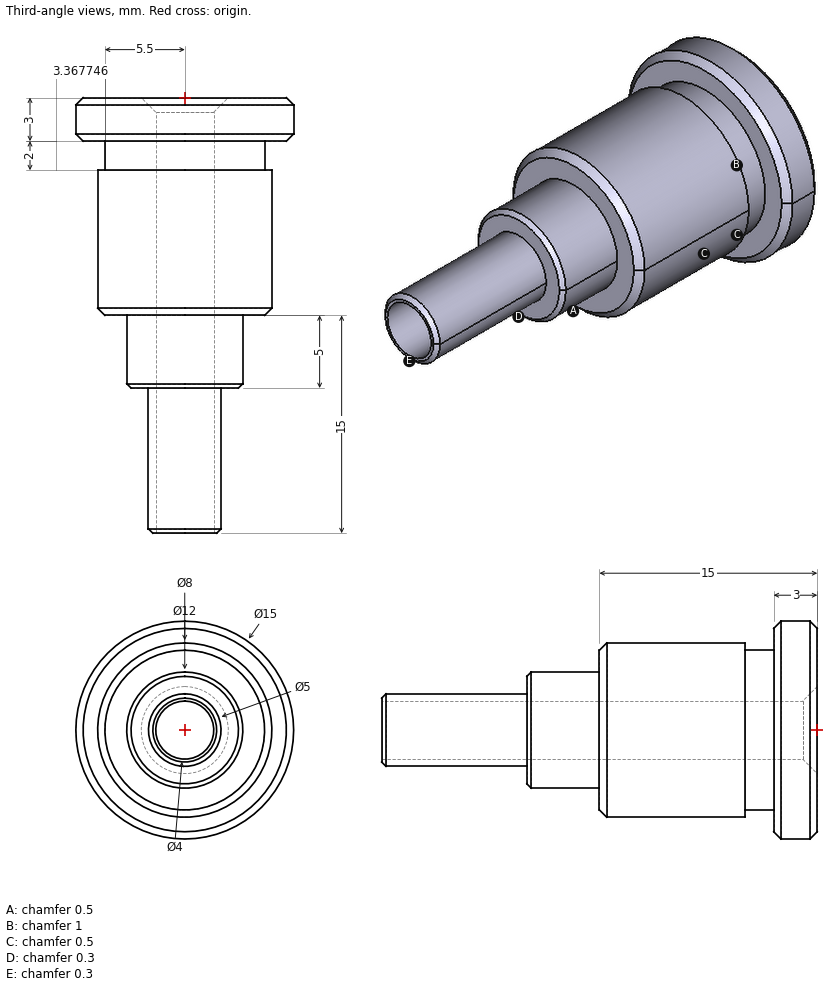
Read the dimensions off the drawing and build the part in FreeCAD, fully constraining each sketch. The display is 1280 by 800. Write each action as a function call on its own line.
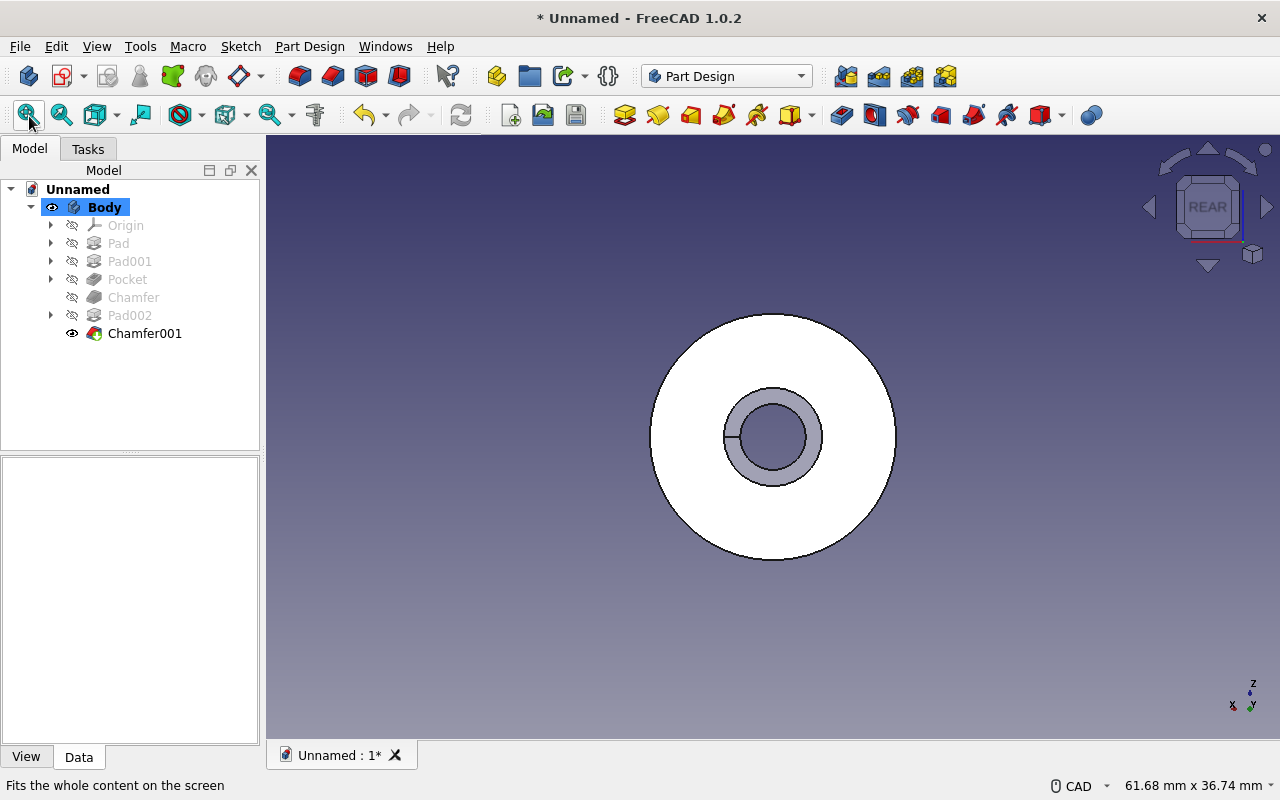
click(896, 436)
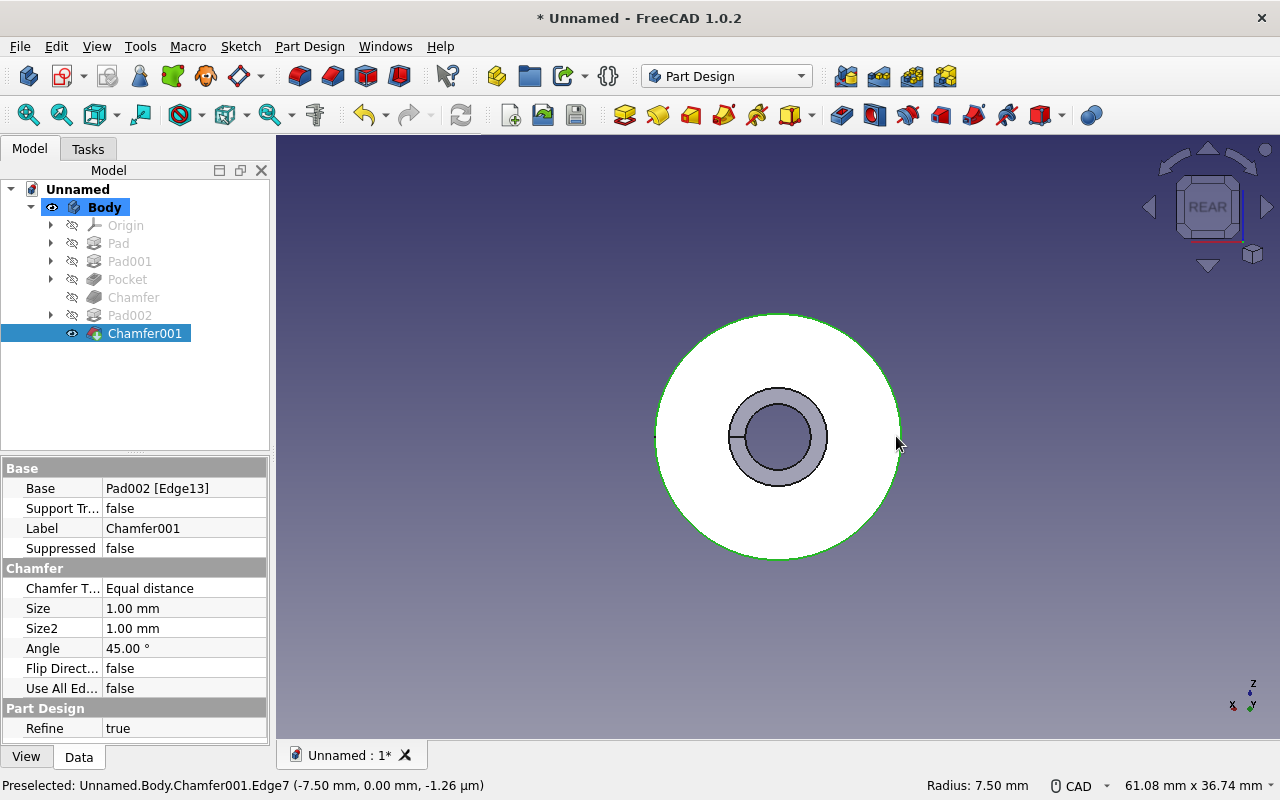
key(0)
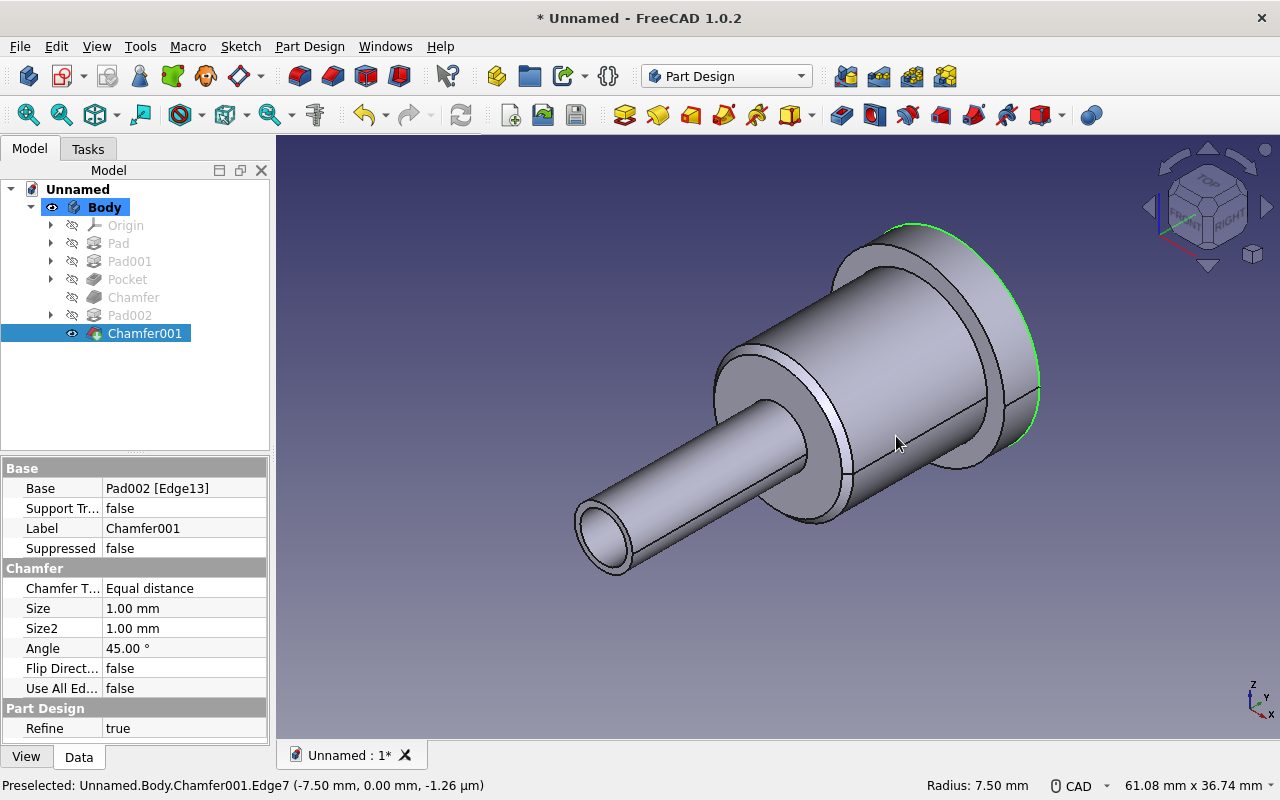
click(891, 244, ctrl)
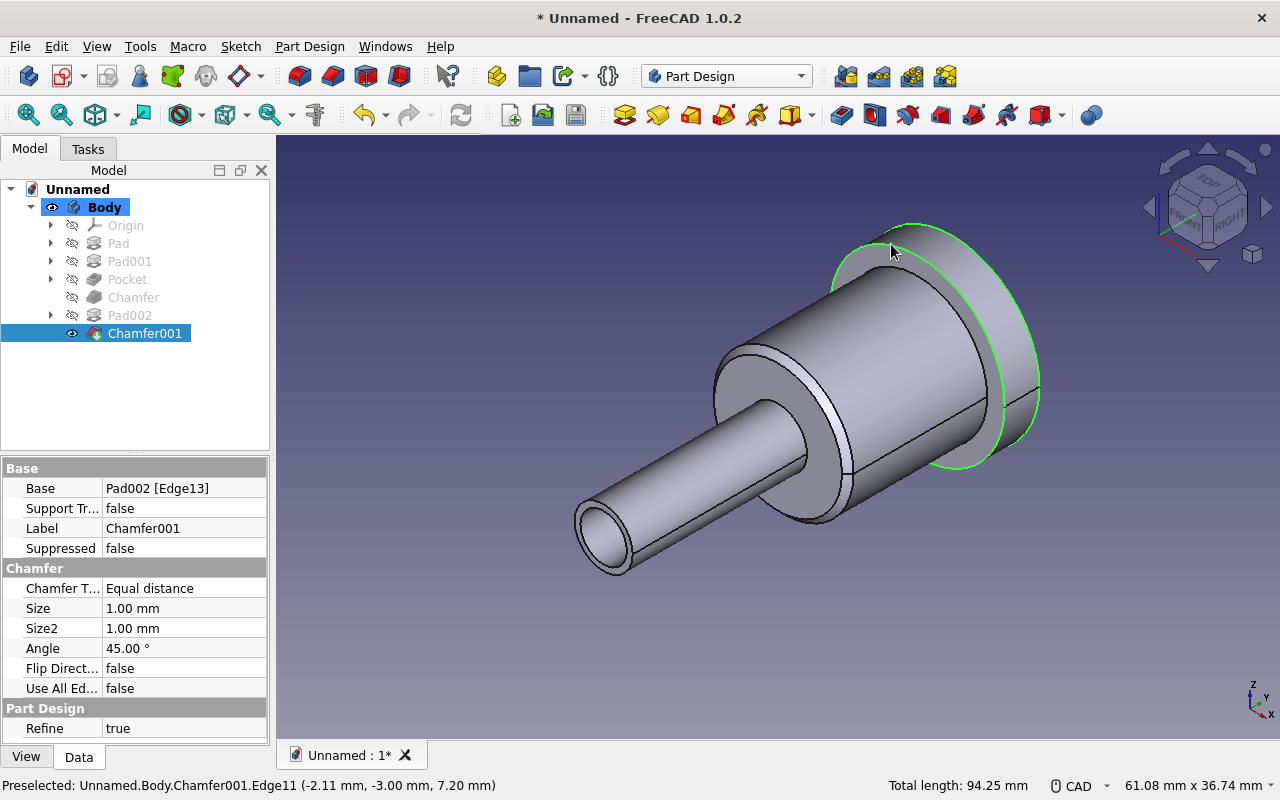
click(333, 76)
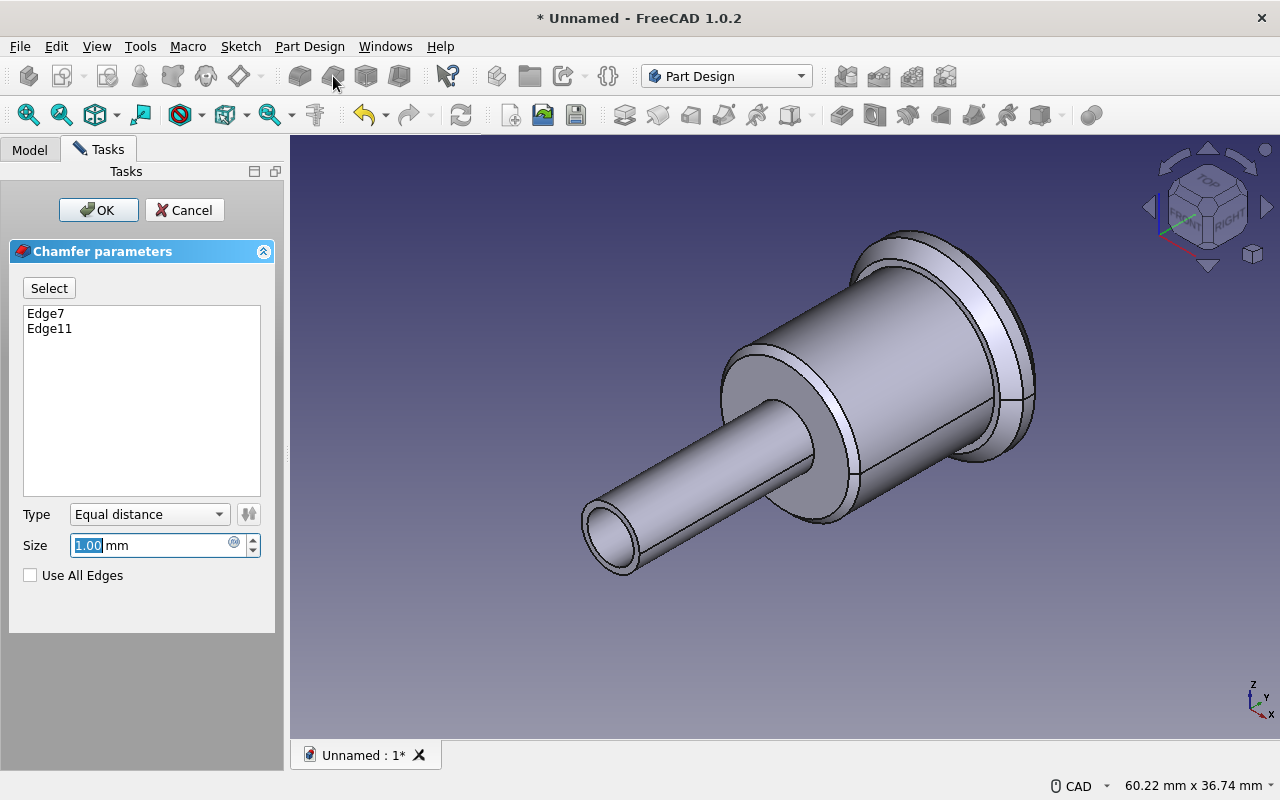
text(0.5)
key(Tab)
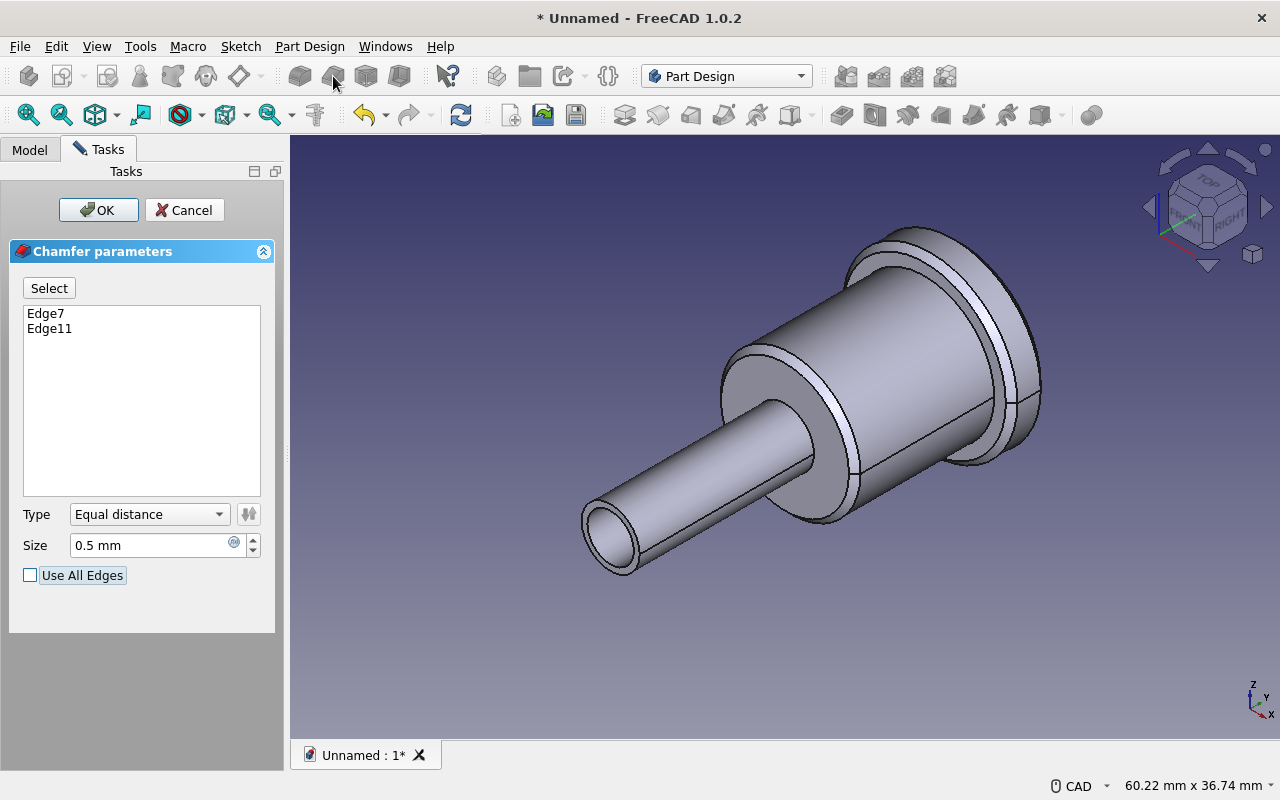
click(99, 210)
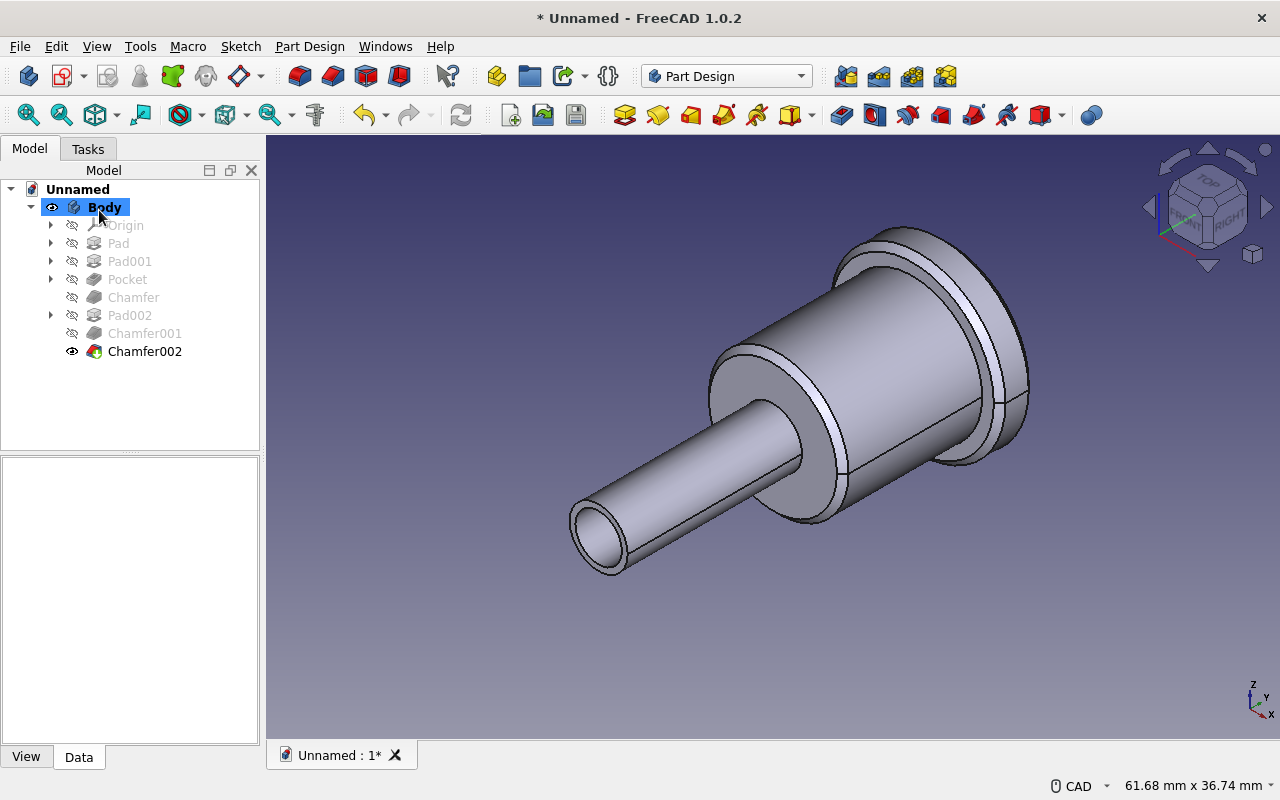
click(810, 499)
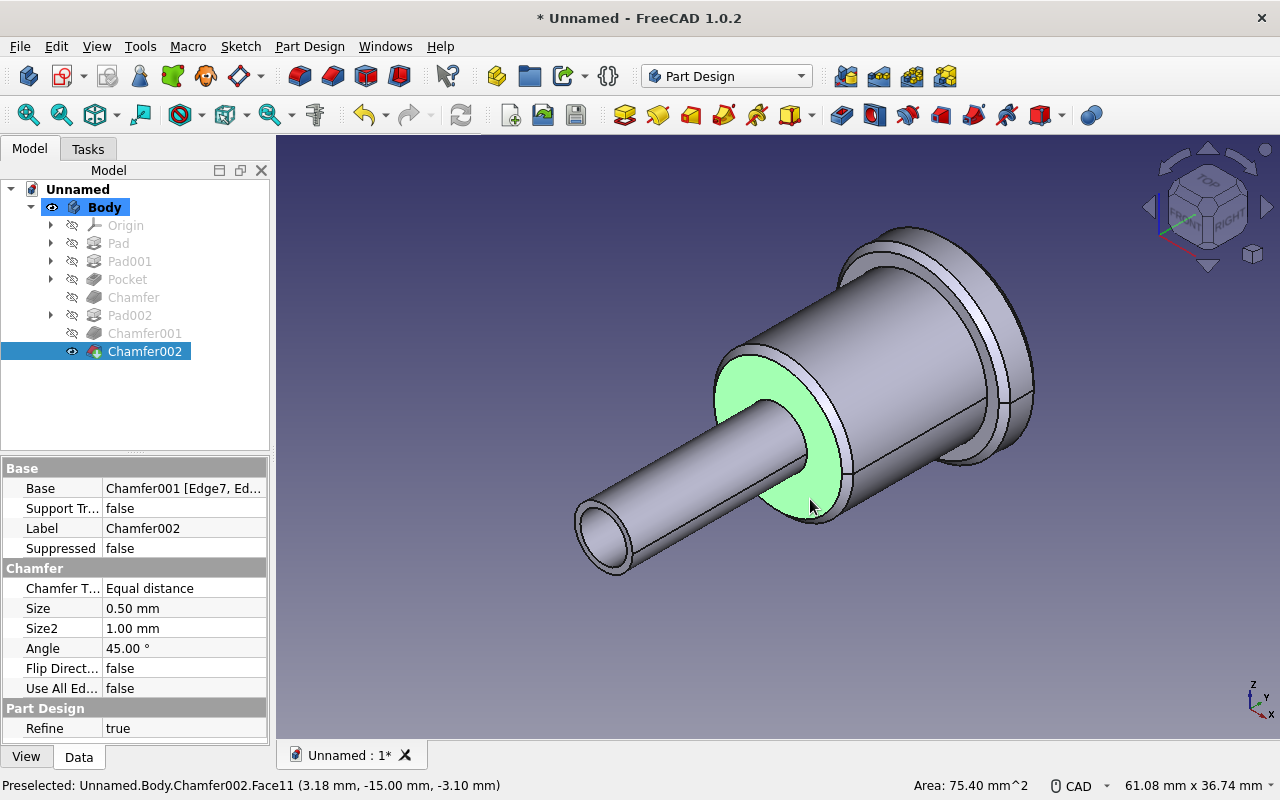
click(62, 76)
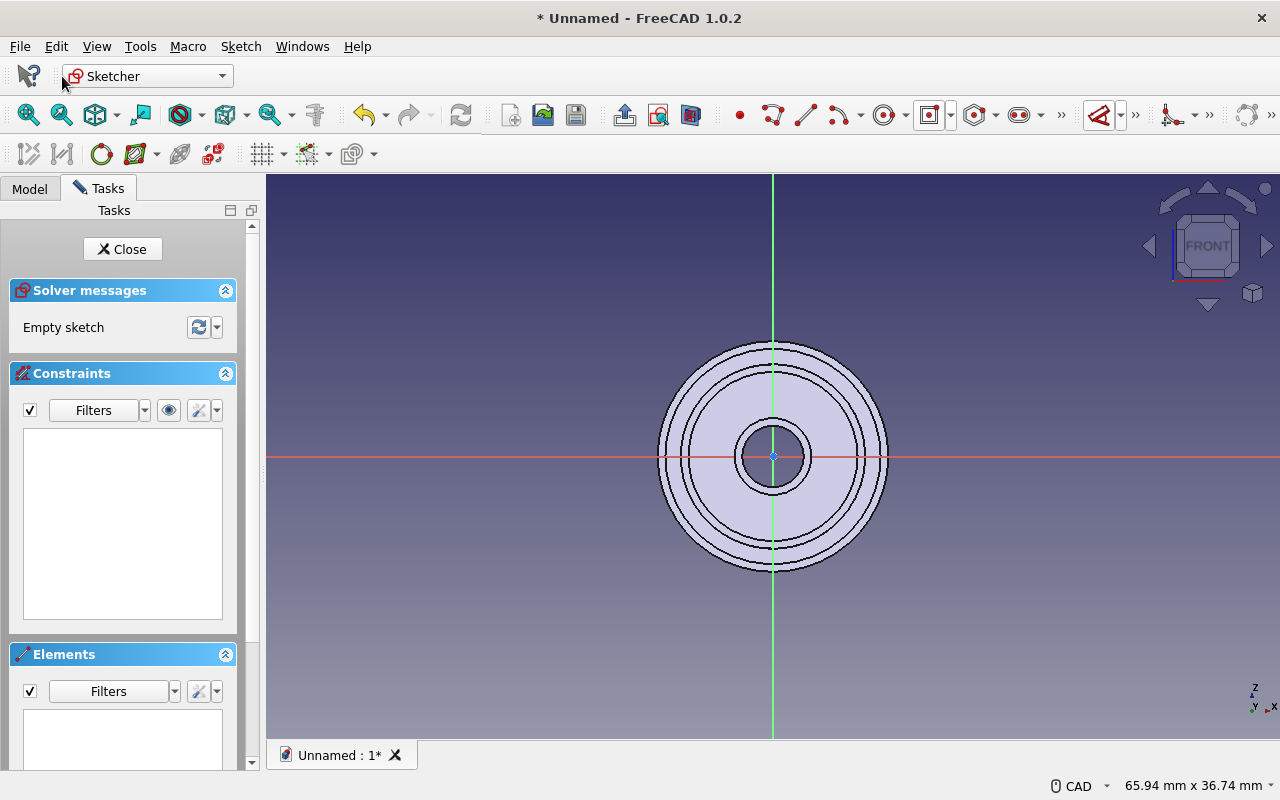
key(q)
key(s)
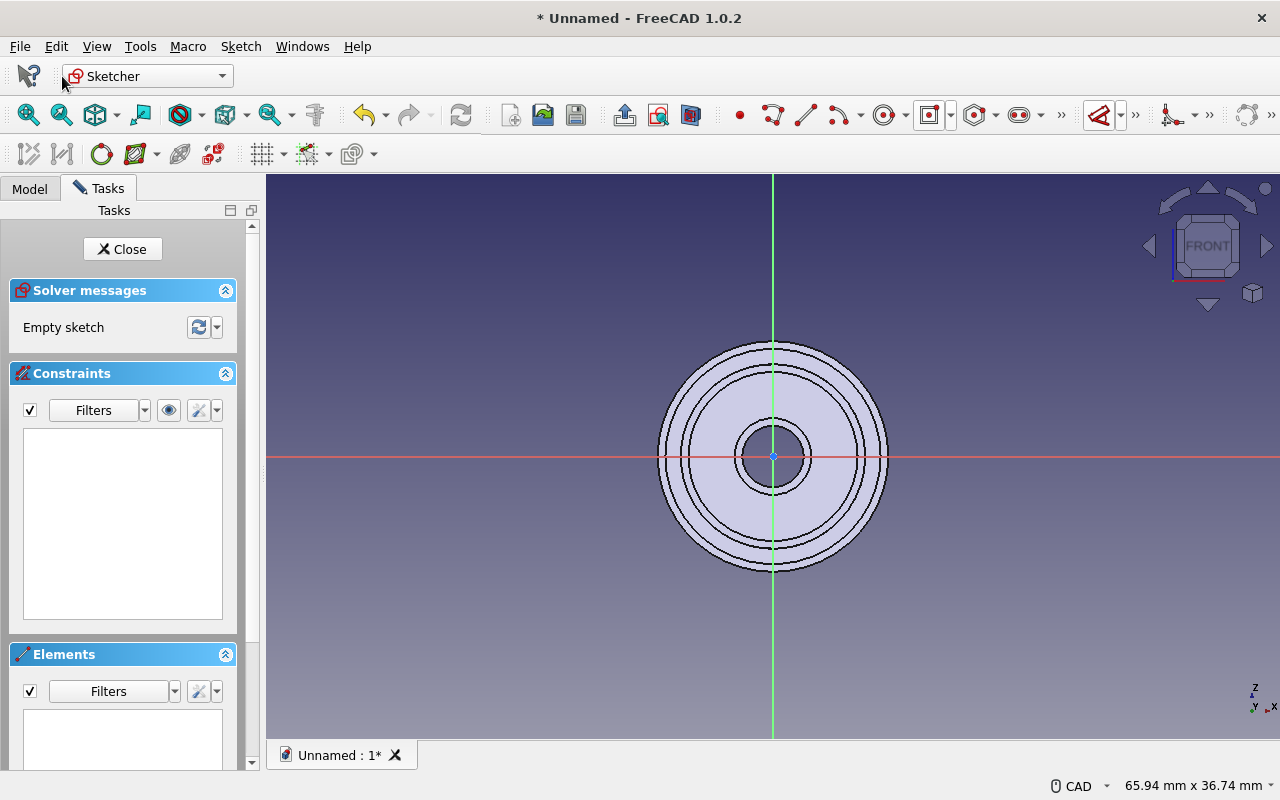
scroll(813, 456, up, 5)